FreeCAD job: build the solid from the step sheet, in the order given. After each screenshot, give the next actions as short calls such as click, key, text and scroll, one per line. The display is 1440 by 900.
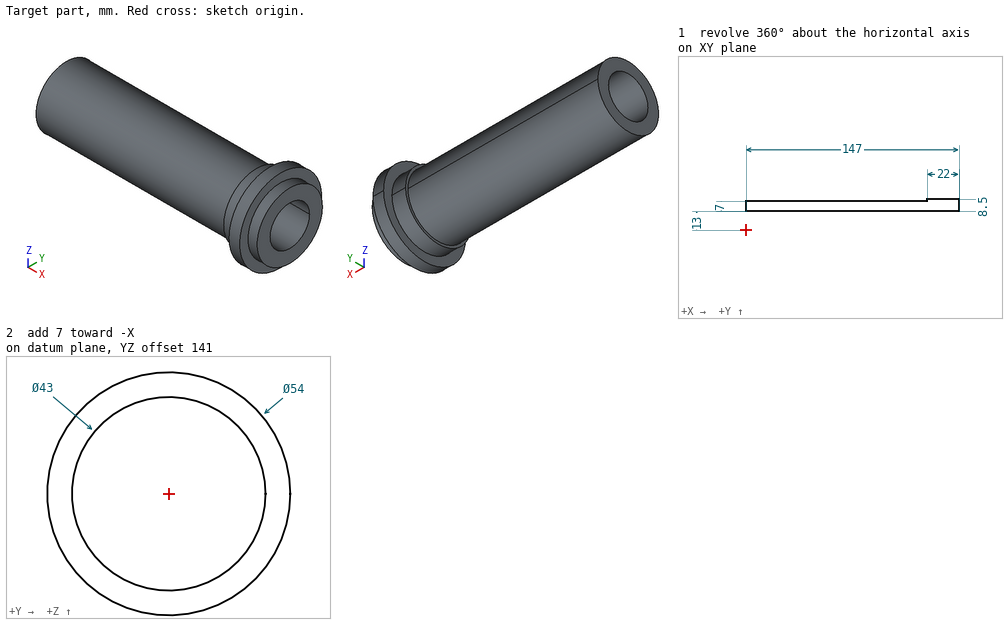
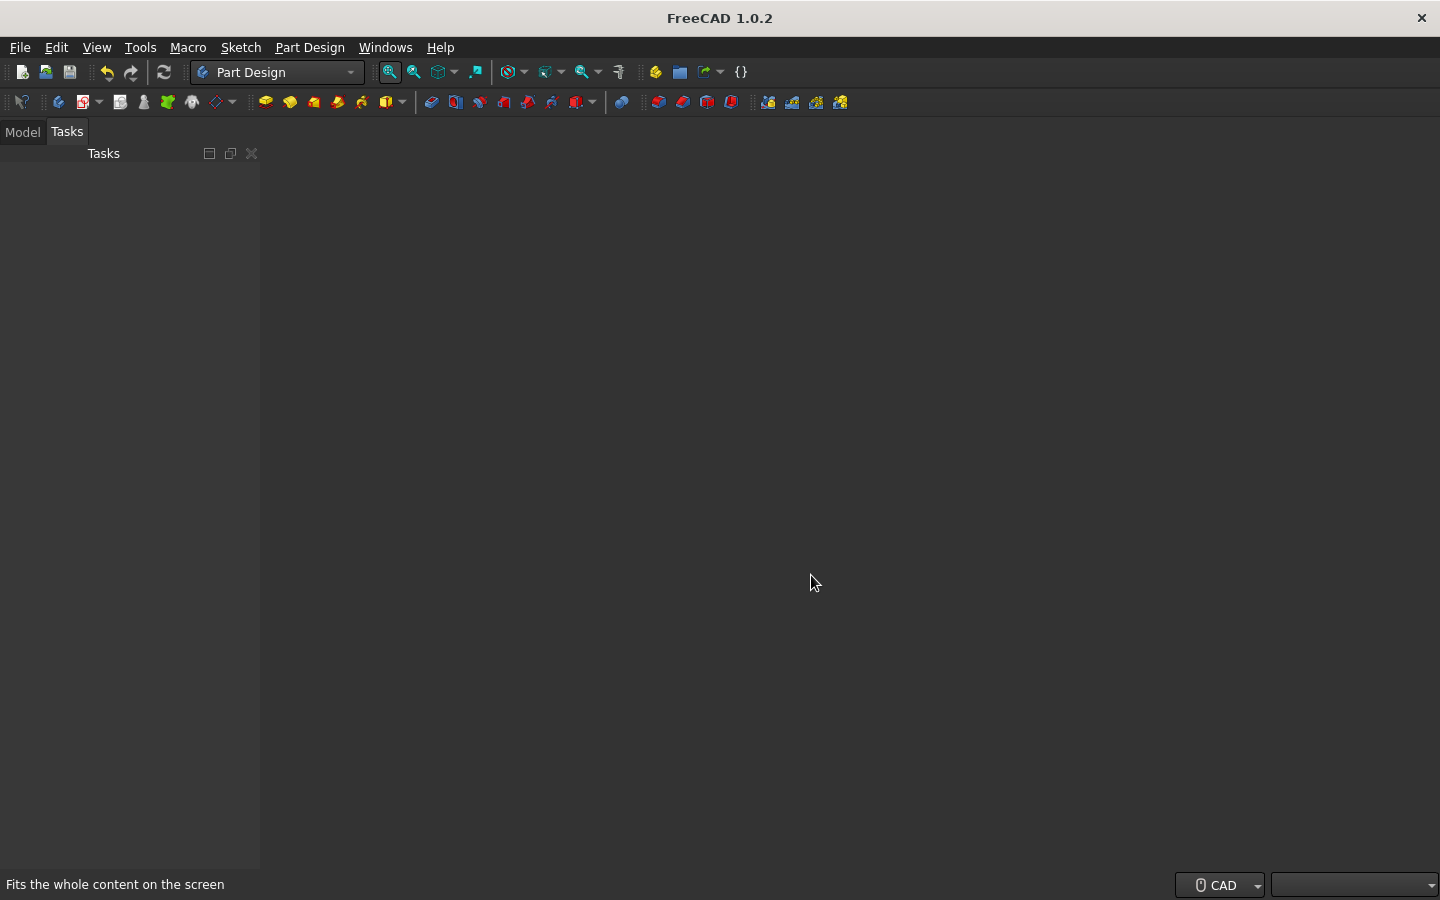
click(22, 72)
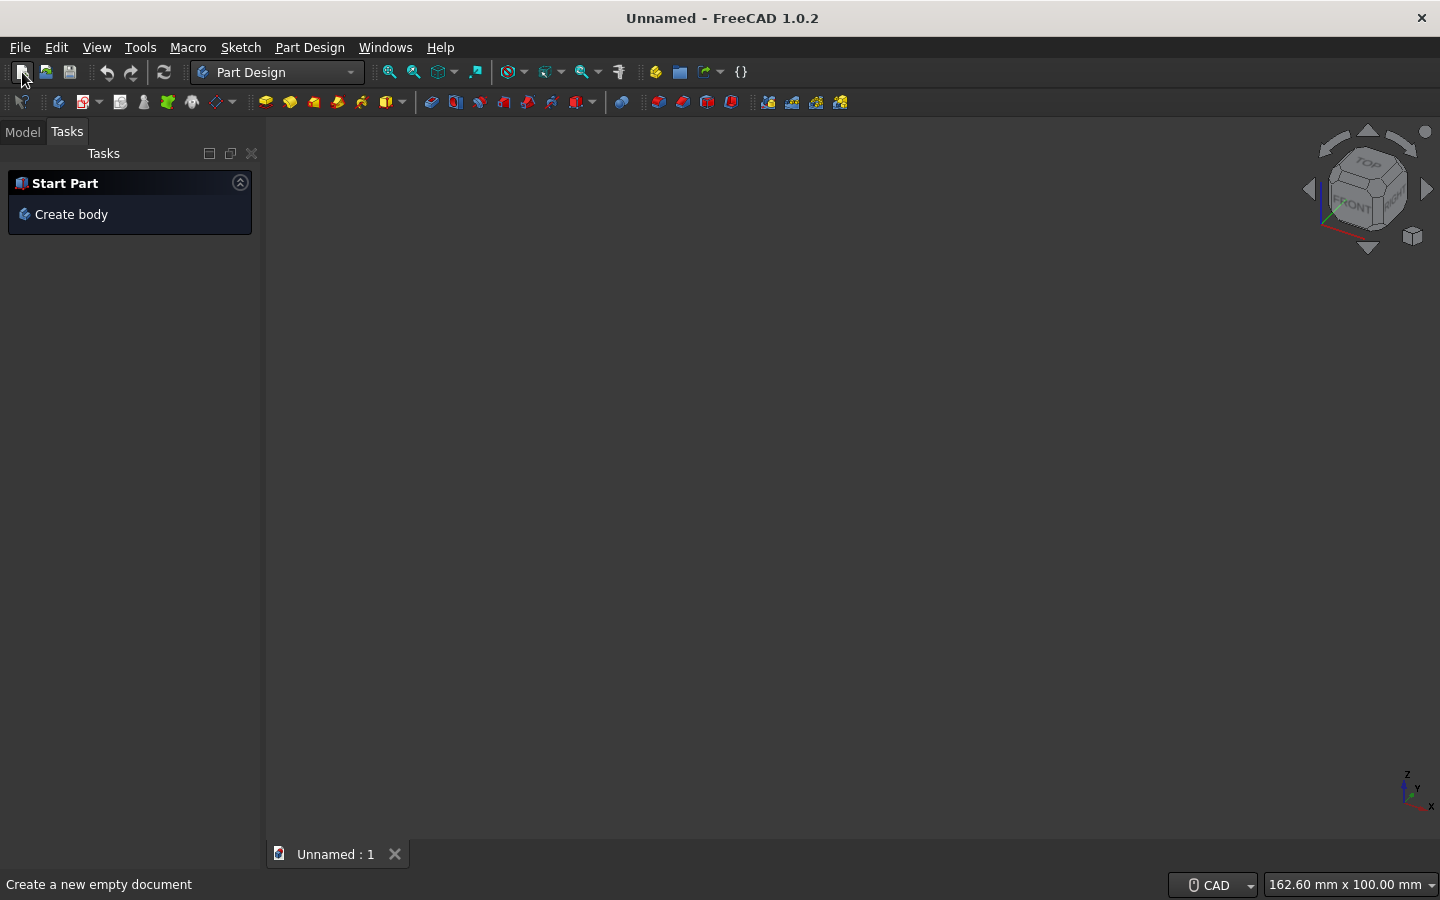
click(84, 102)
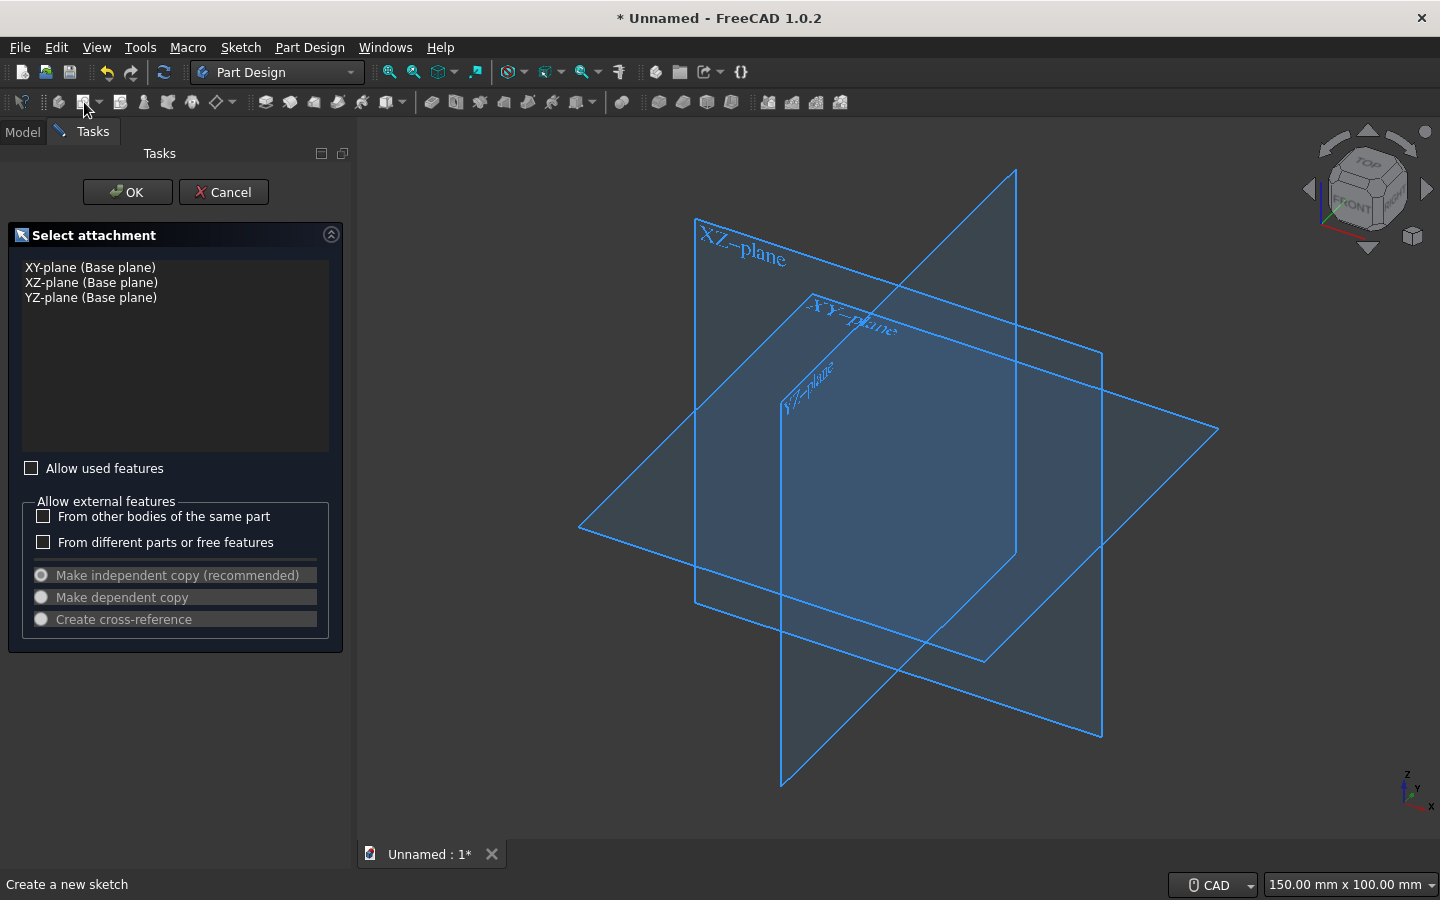
click(82, 268)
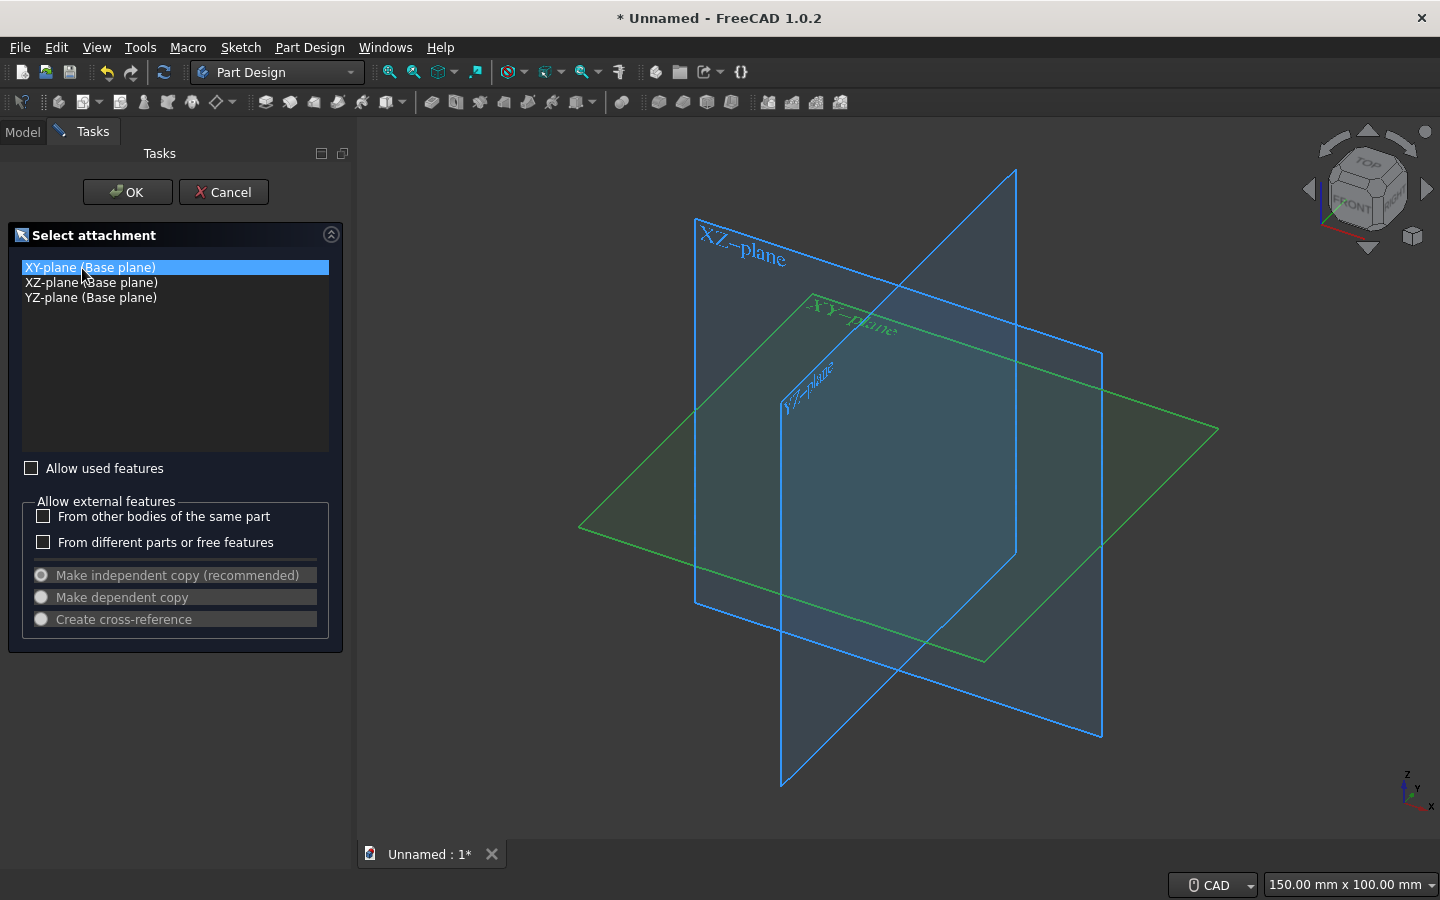
click(128, 192)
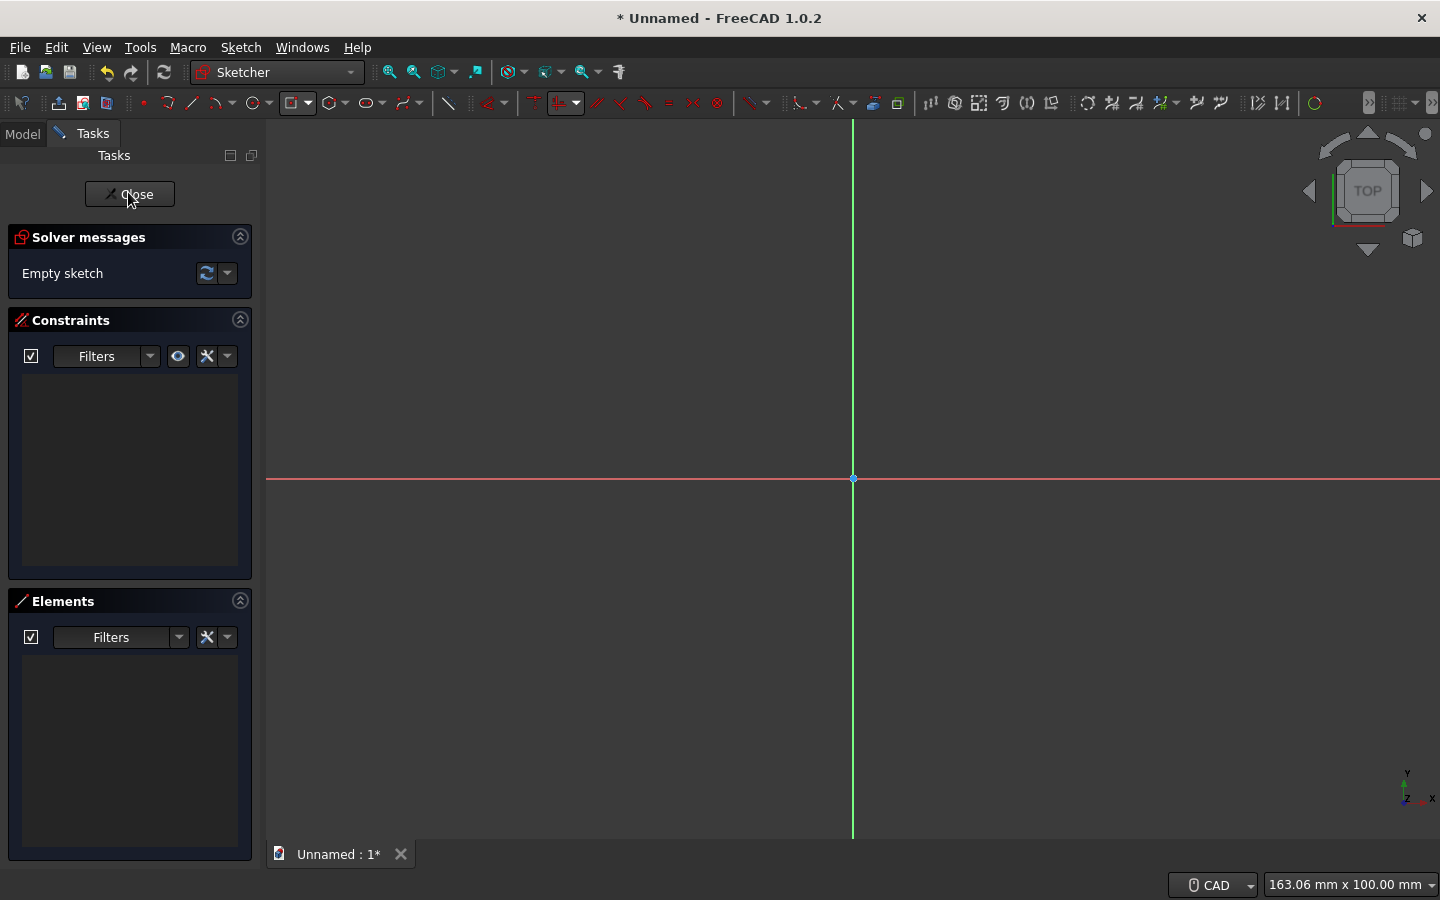
scroll(294, 573, down, 3)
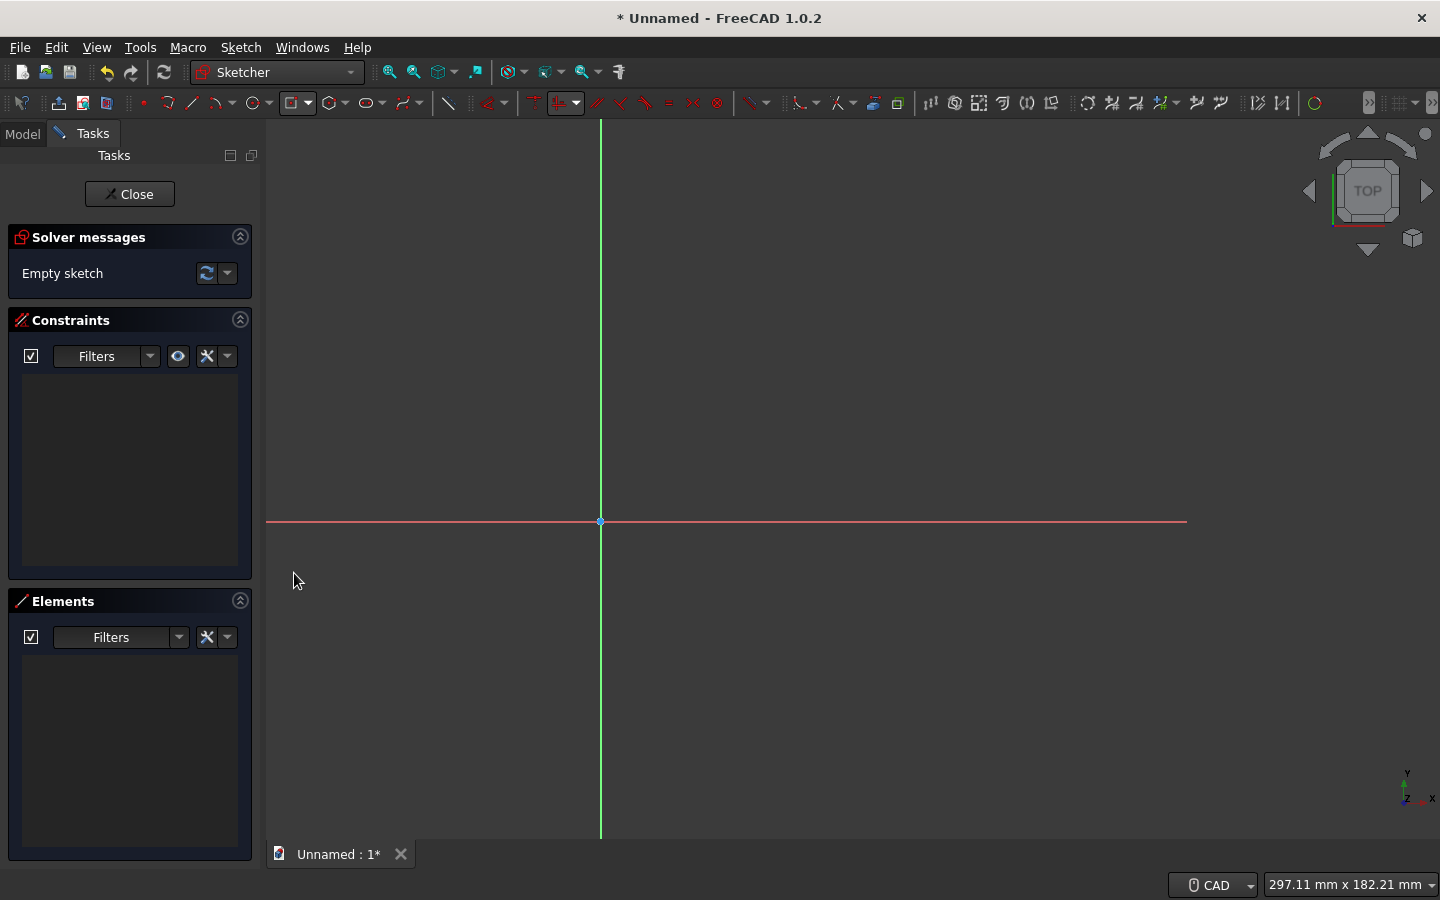
click(168, 104)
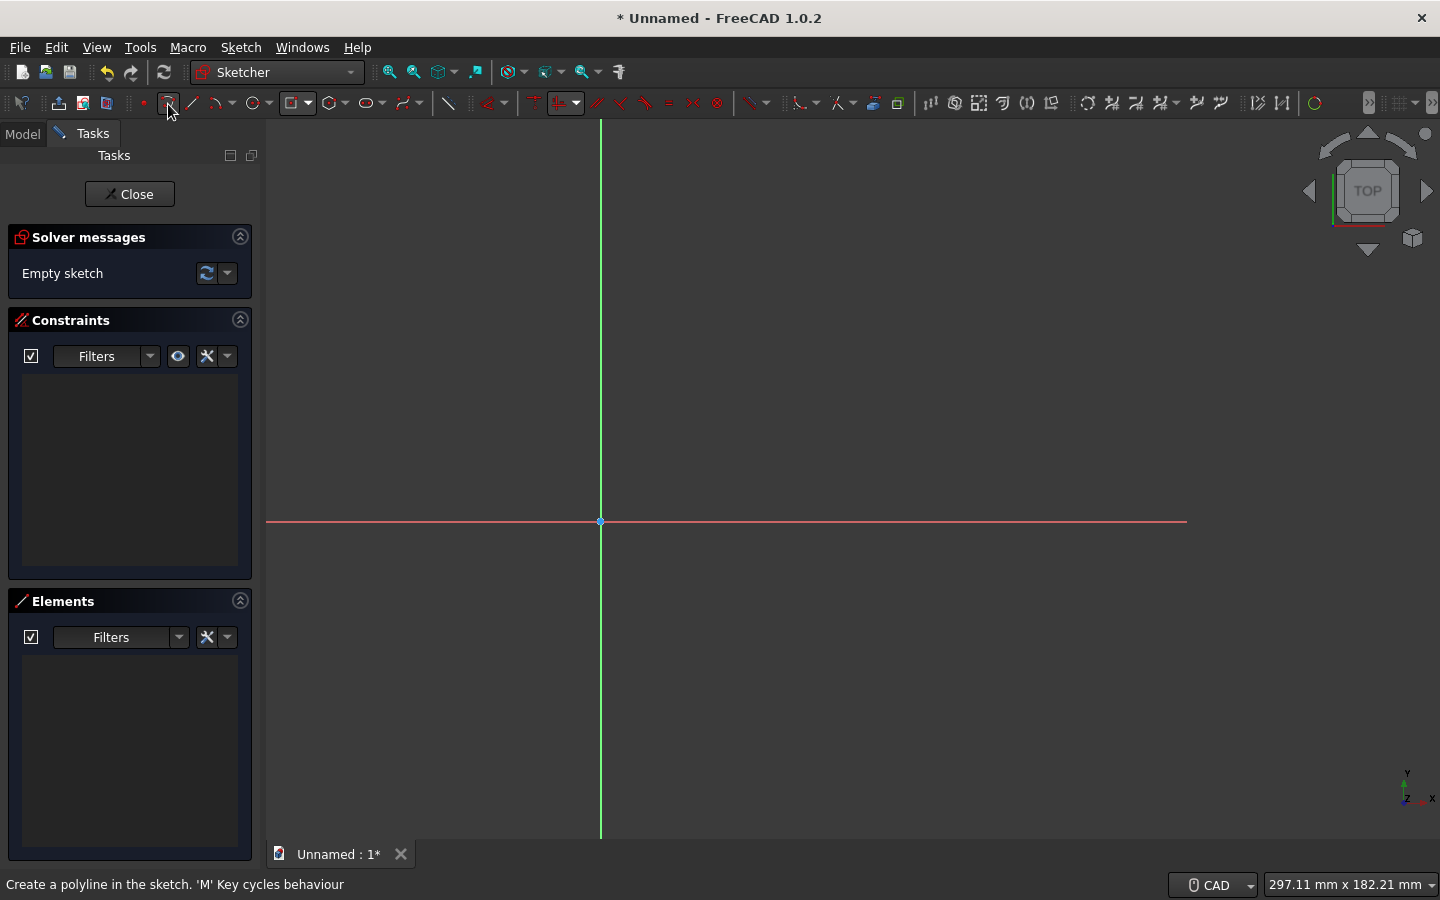
click(601, 470)
click(1182, 470)
click(1182, 437)
click(1095, 437)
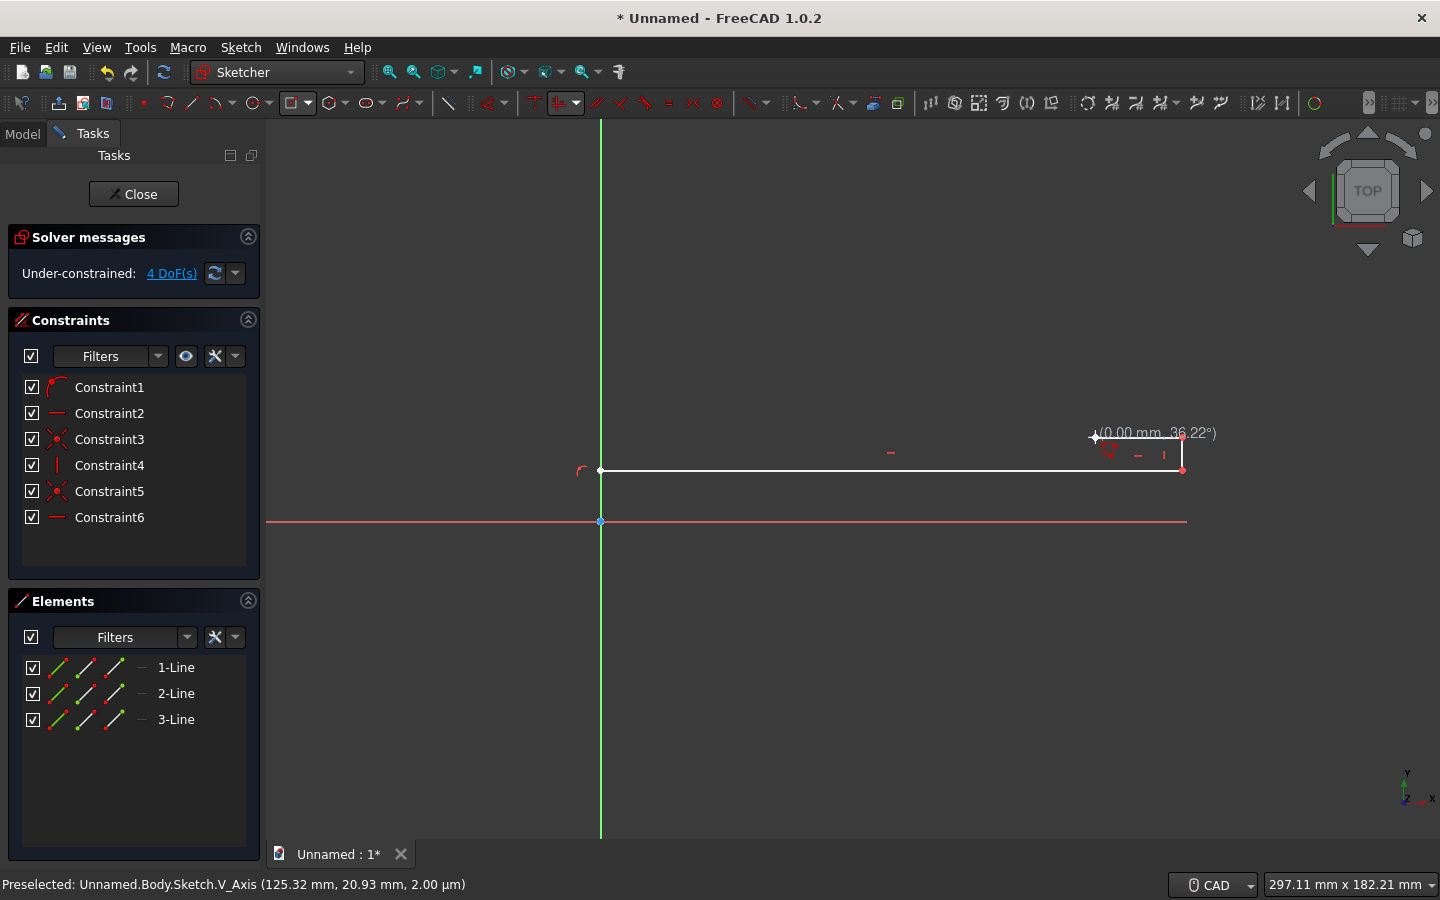
scroll(1095, 443, up, 5)